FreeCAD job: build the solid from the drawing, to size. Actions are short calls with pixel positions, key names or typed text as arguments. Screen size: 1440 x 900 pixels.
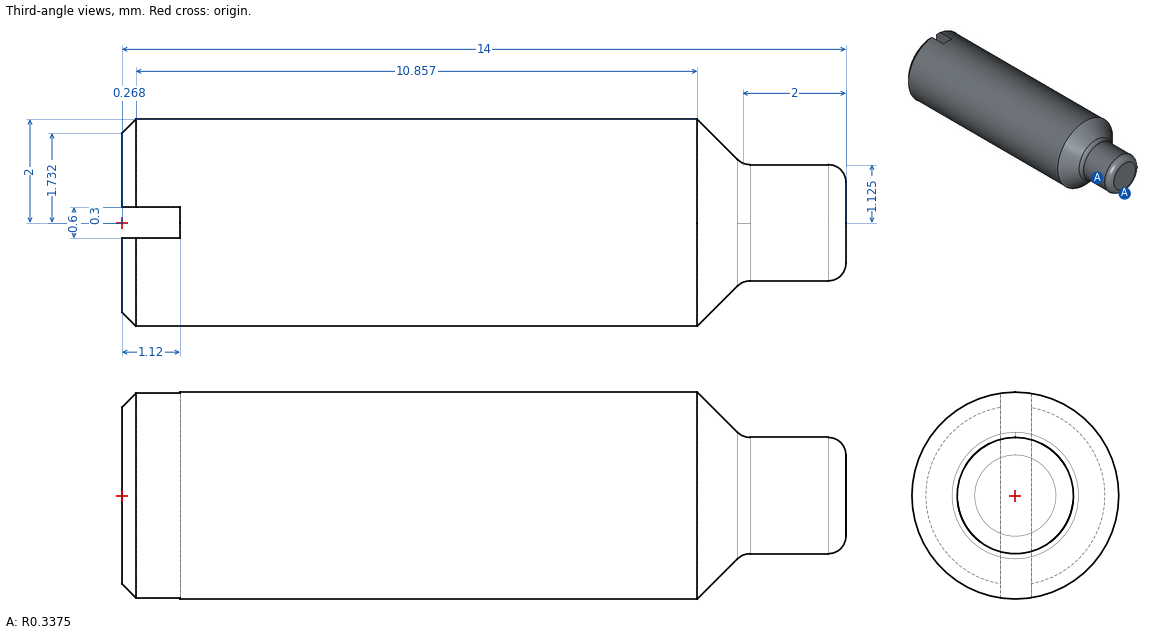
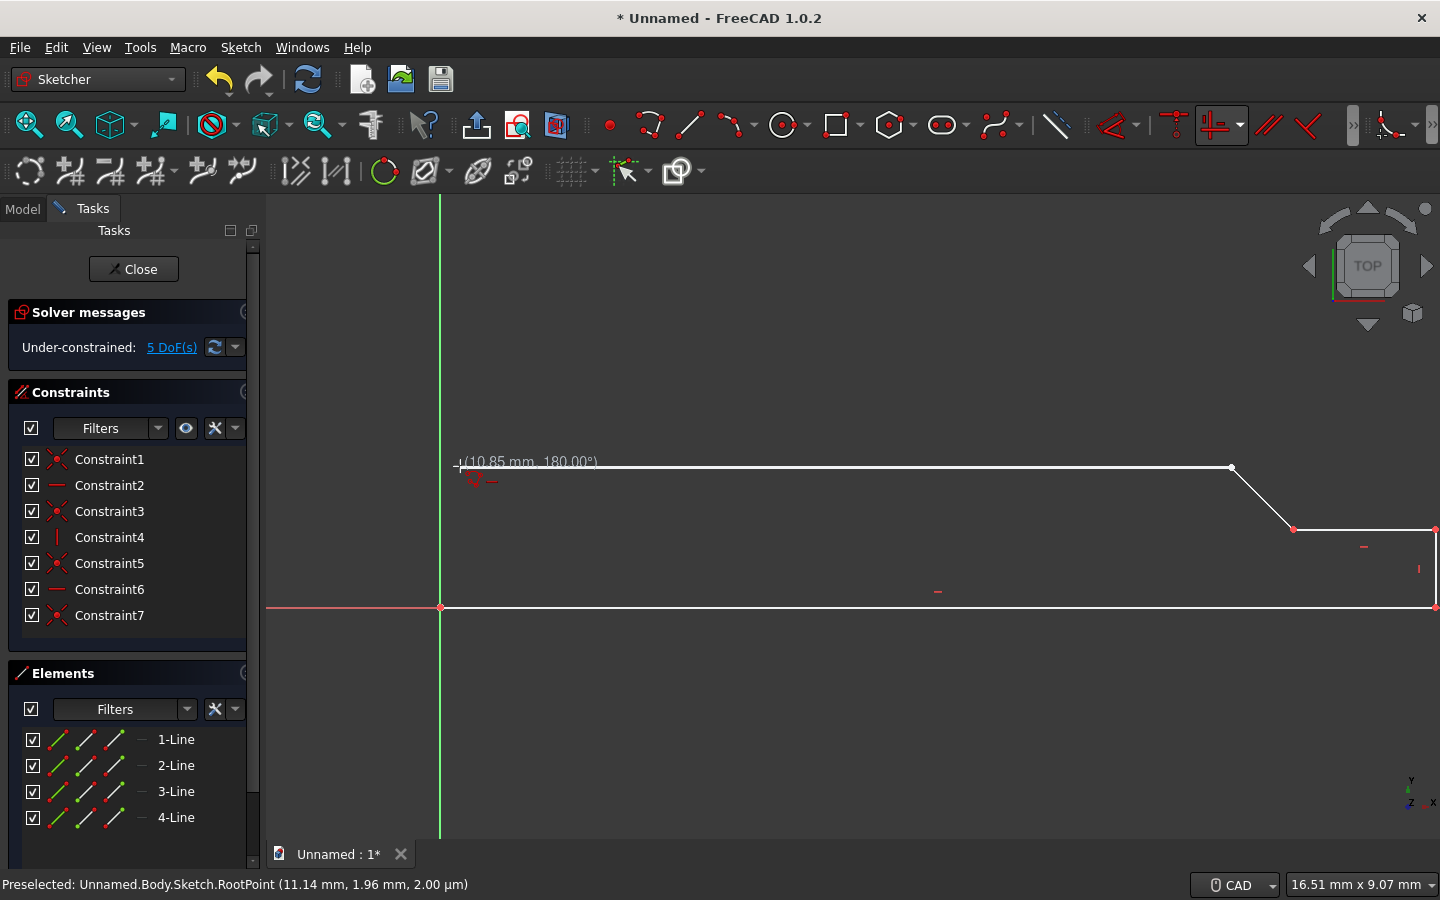
click(460, 466)
click(449, 485)
click(440, 608)
key(Escape)
key(Escape)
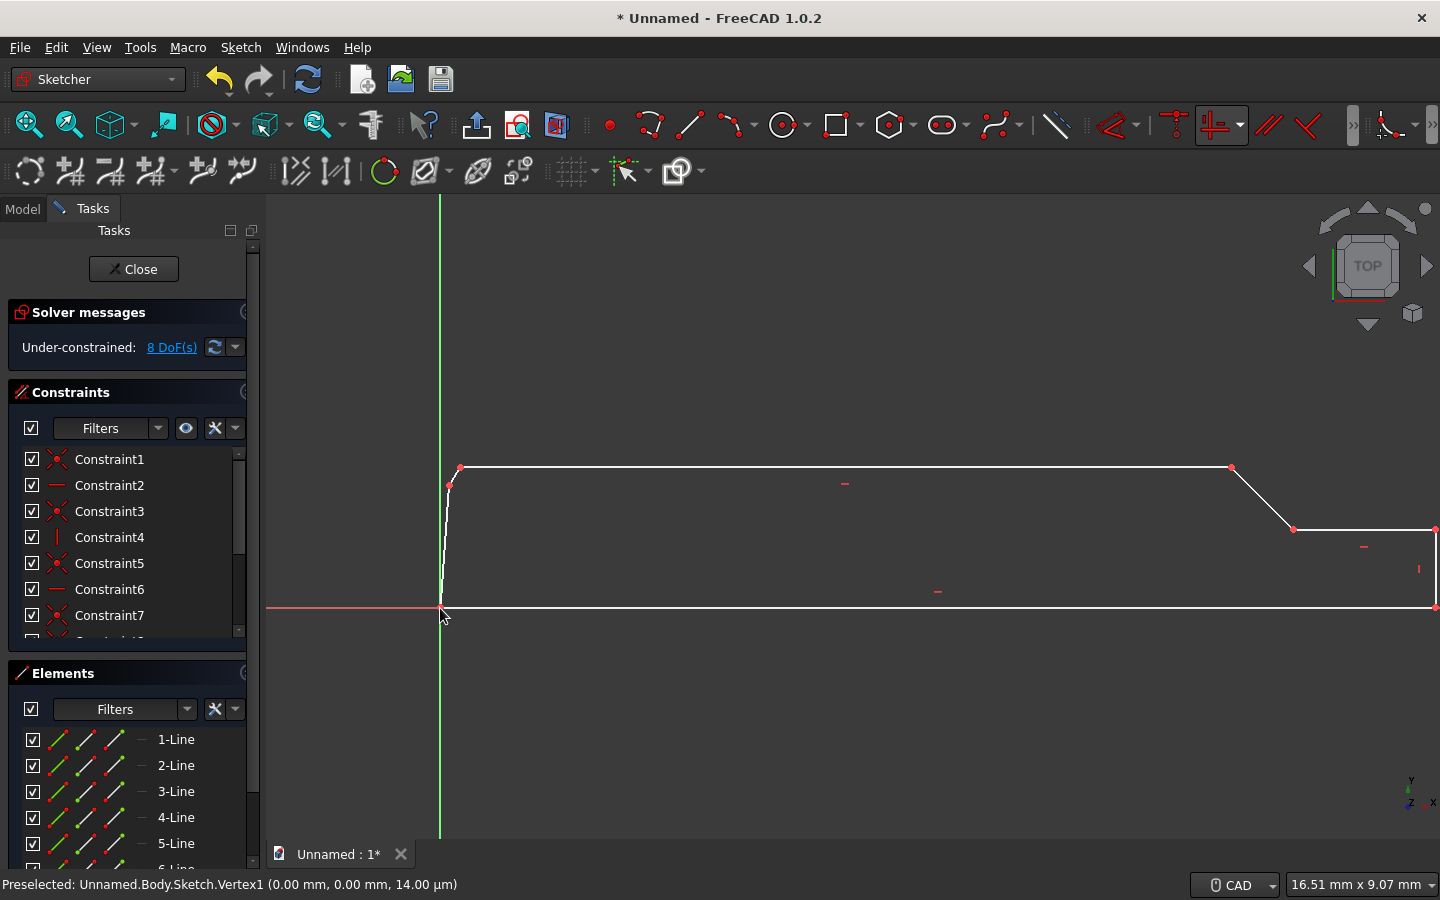
click(443, 571)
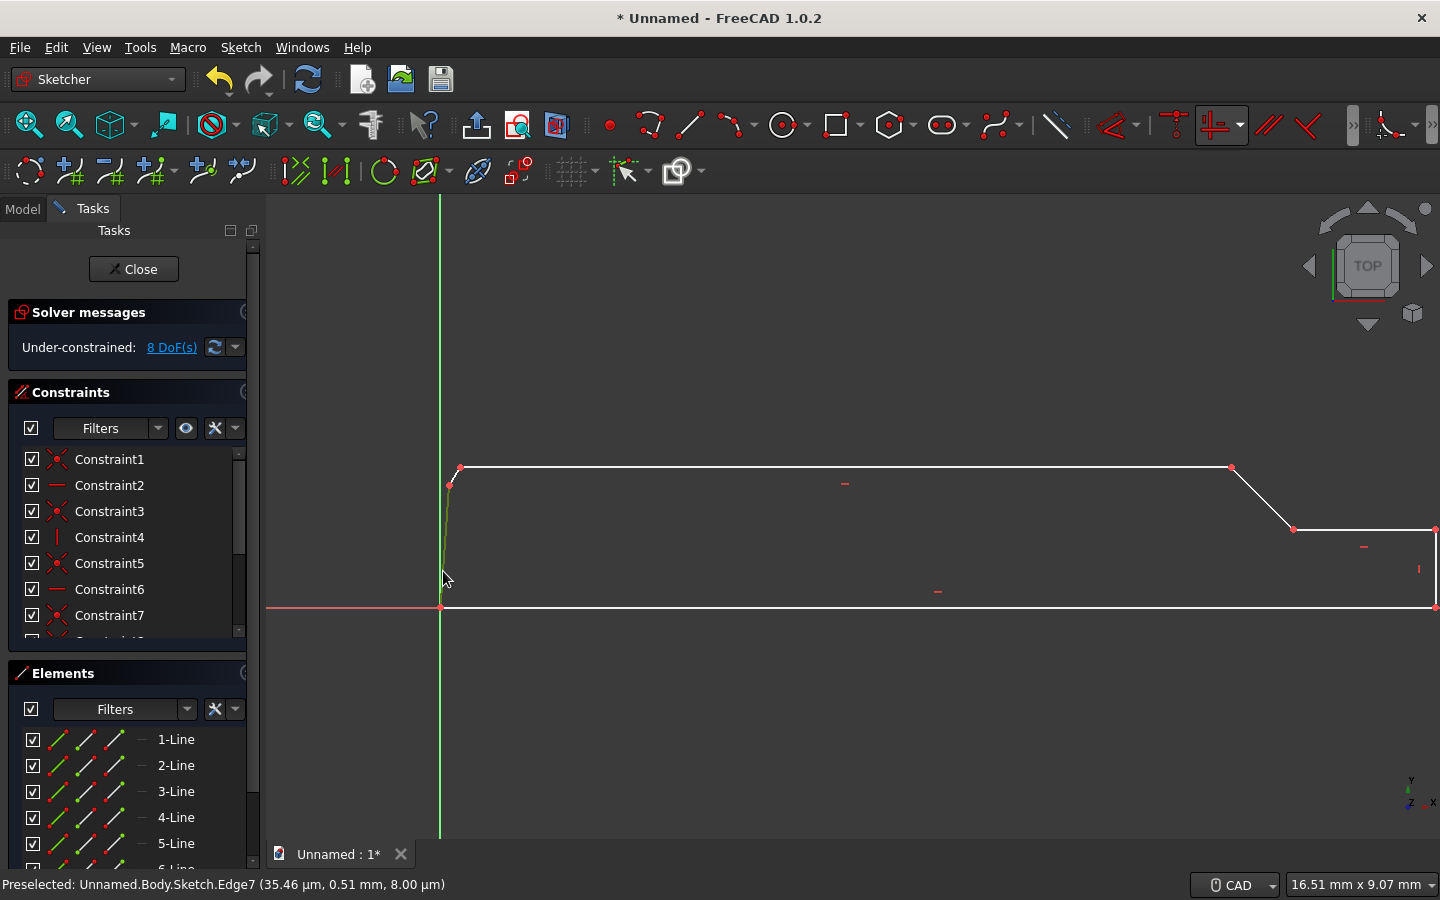
key(v)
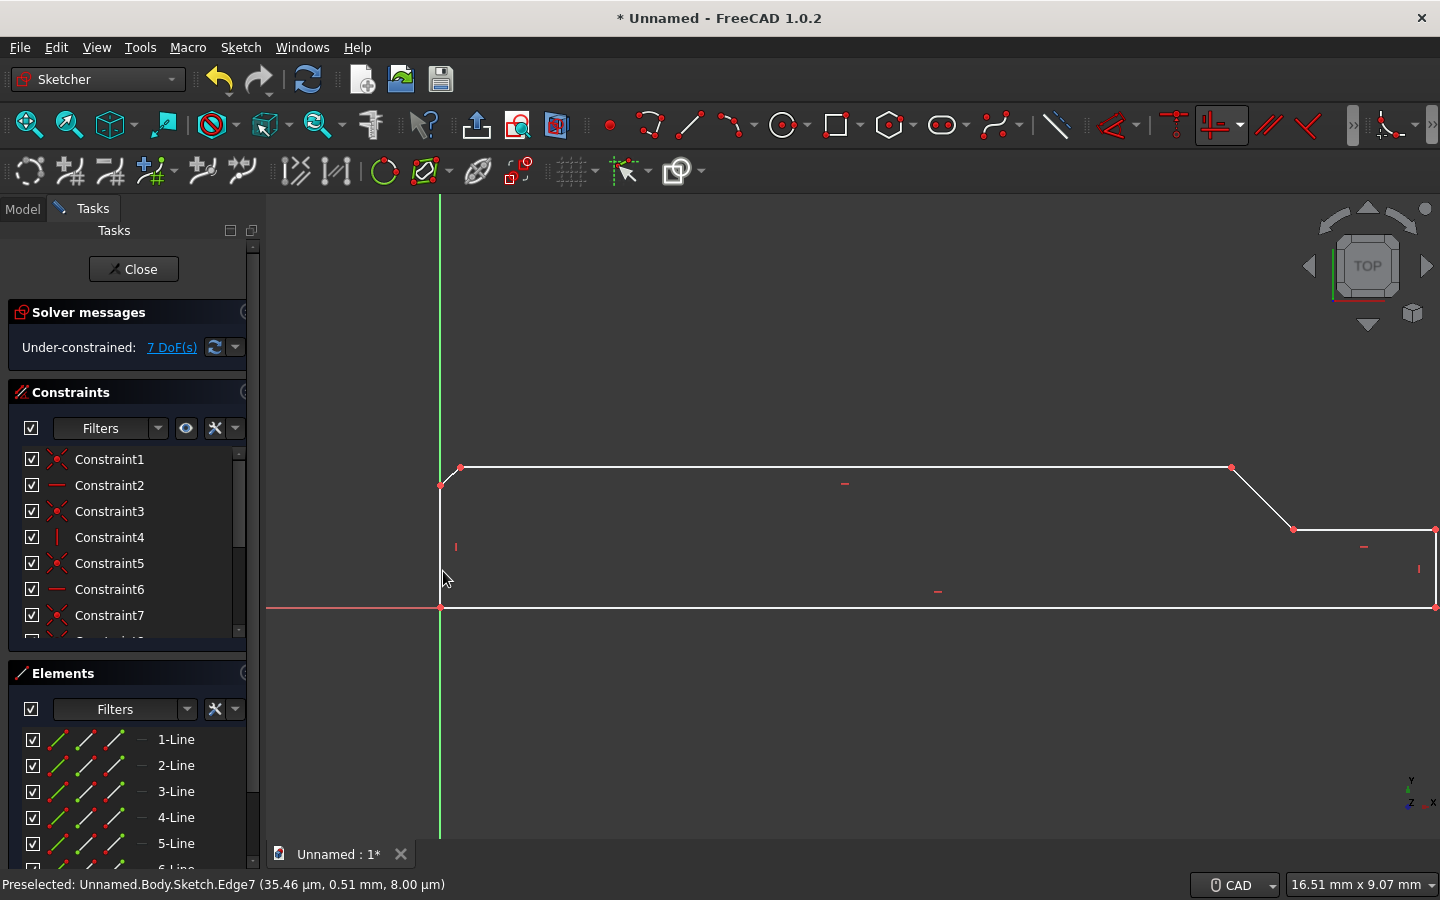
key(d)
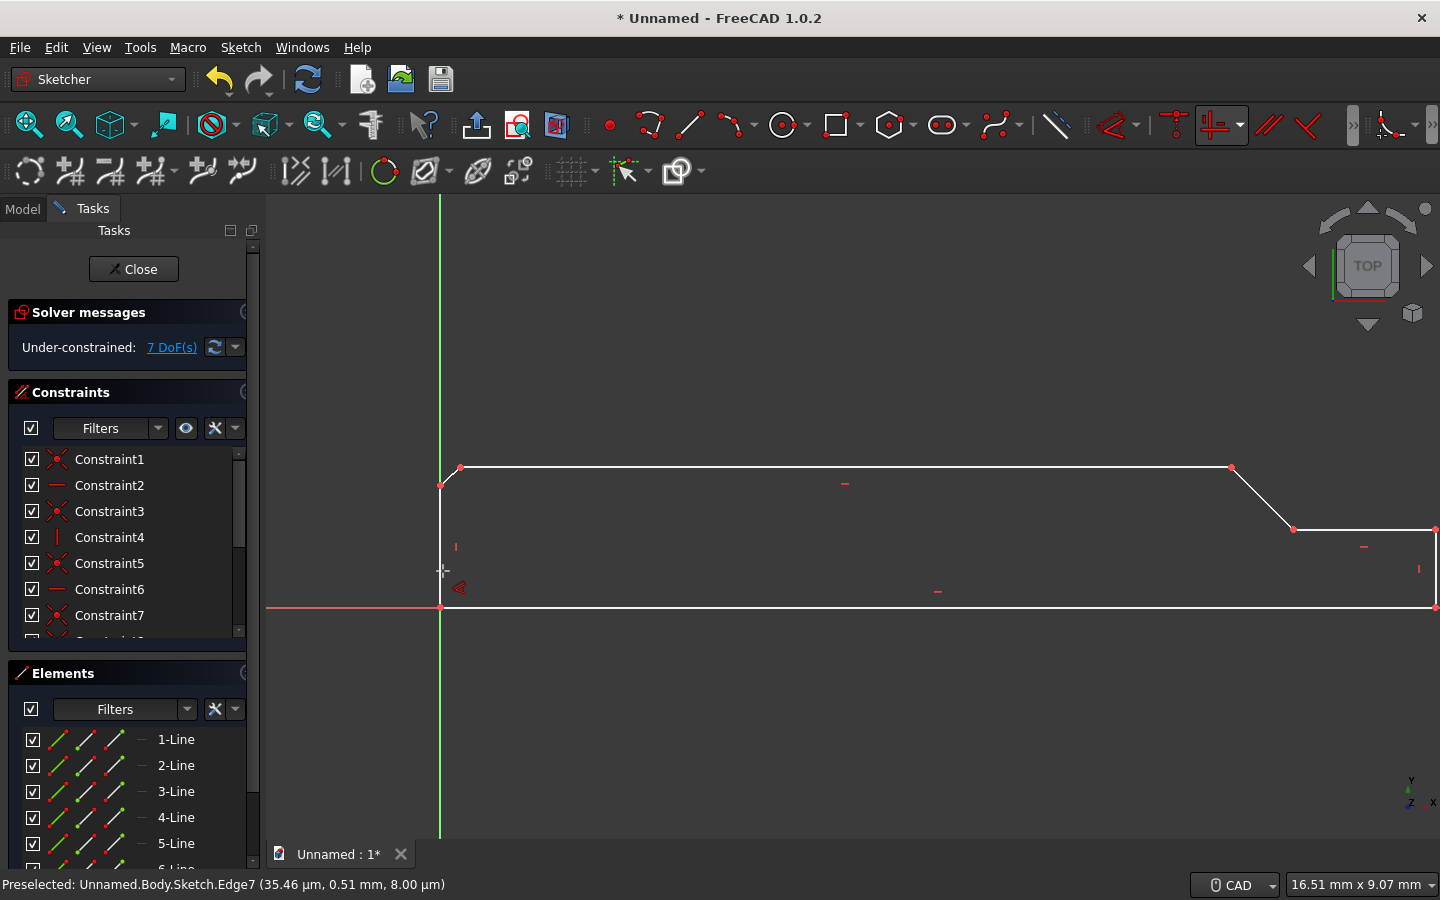
scroll(472, 475, down, 2)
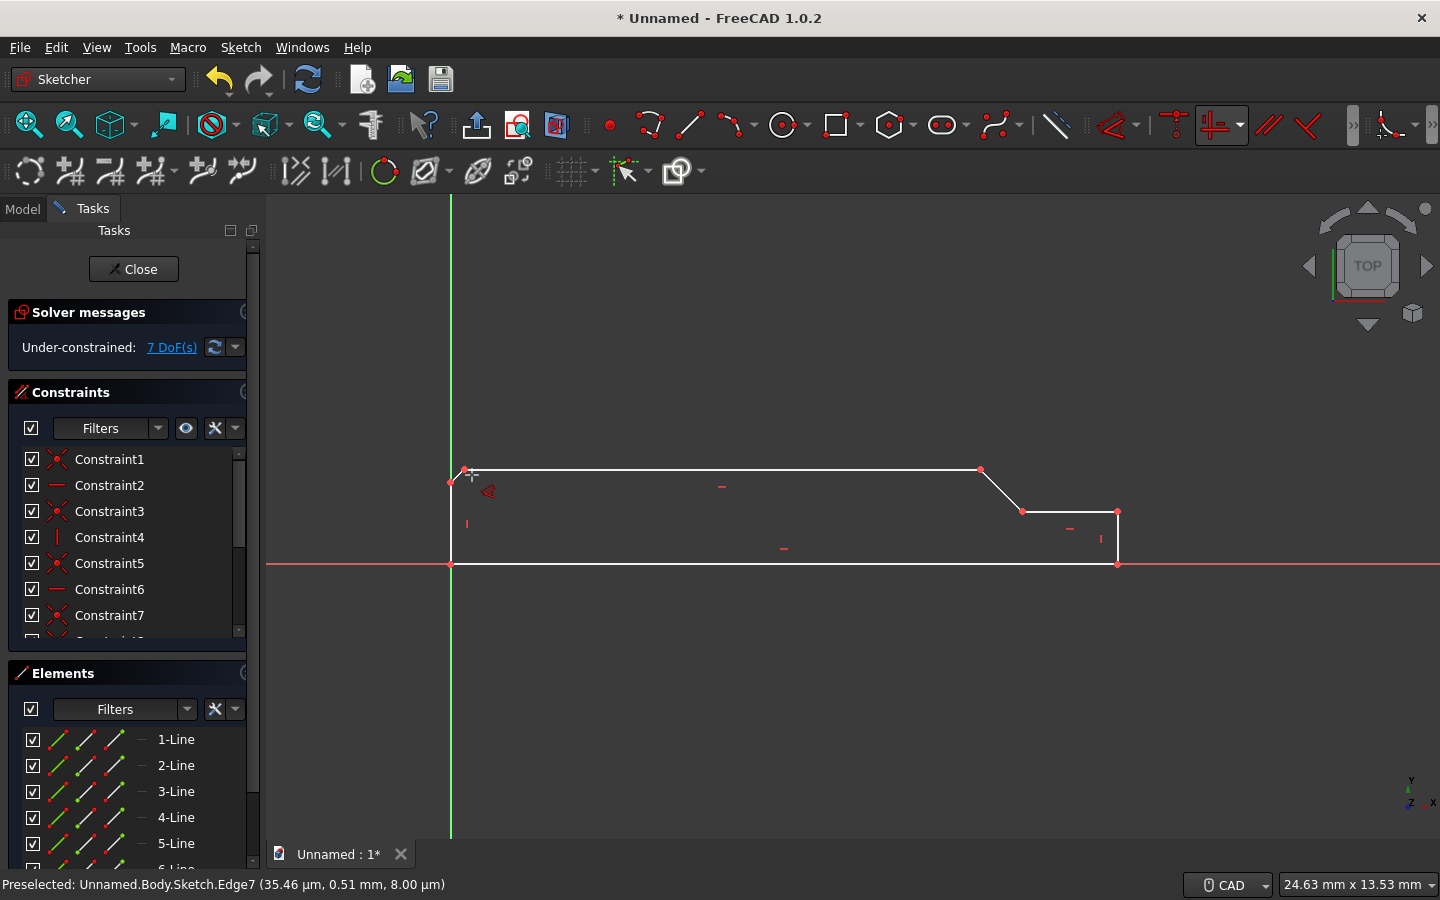
click(1089, 512)
click(1070, 478)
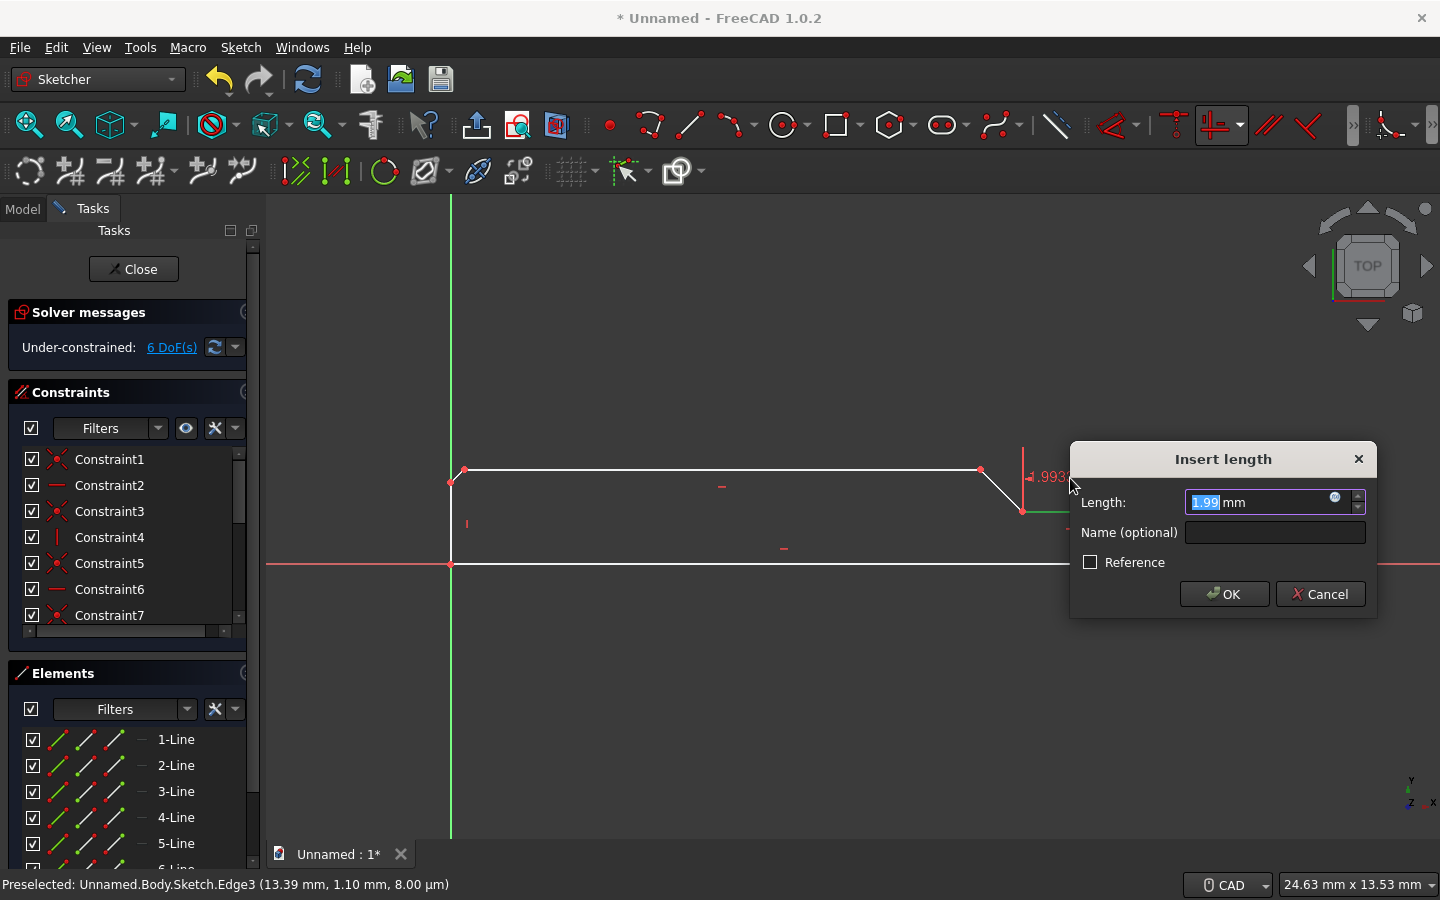
text(2)
key(Return)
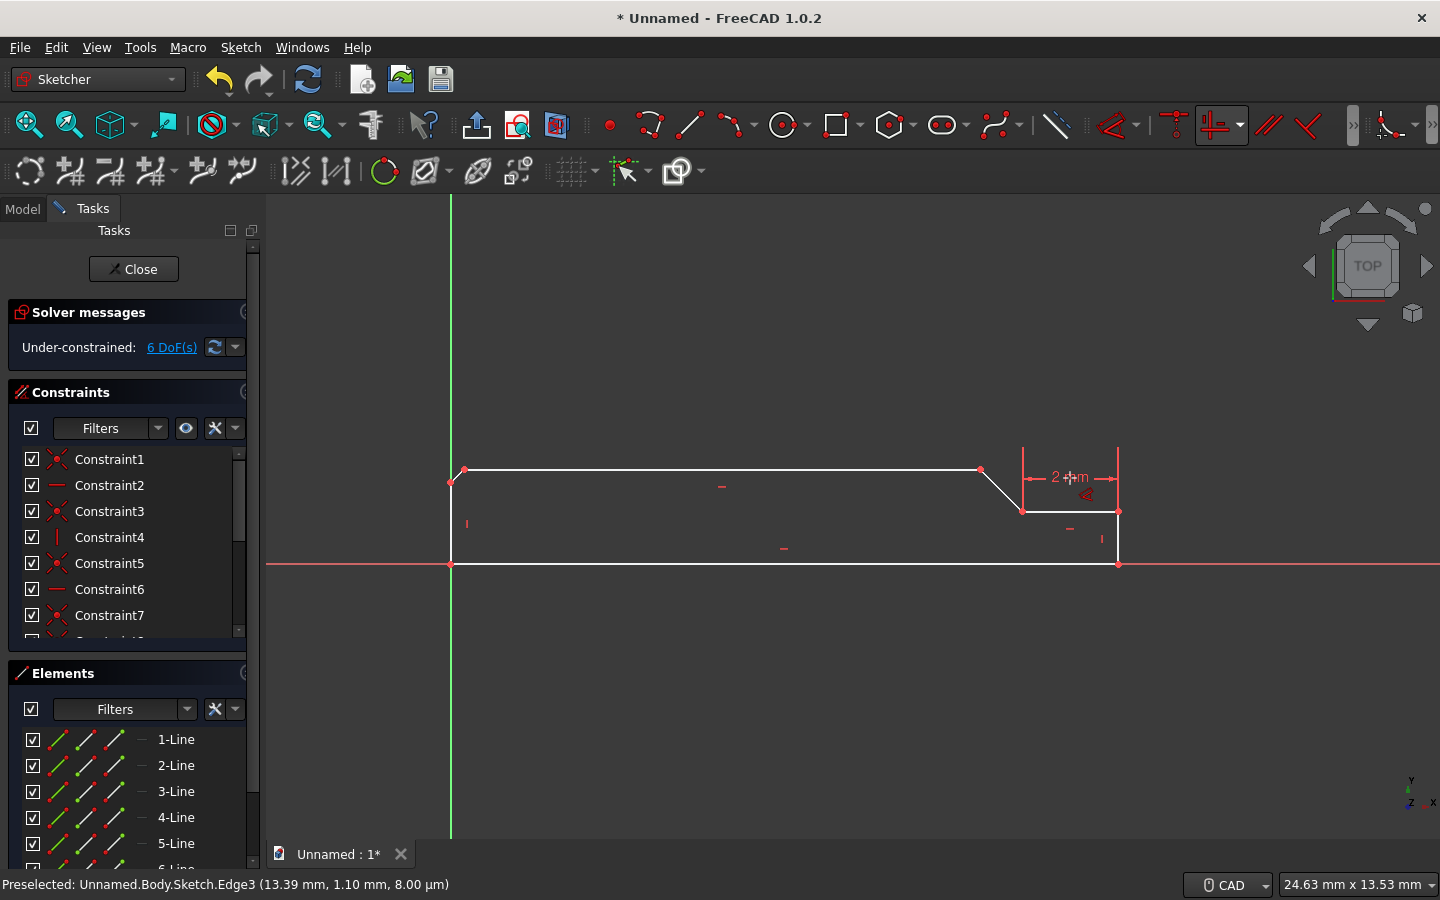
click(651, 564)
click(785, 598)